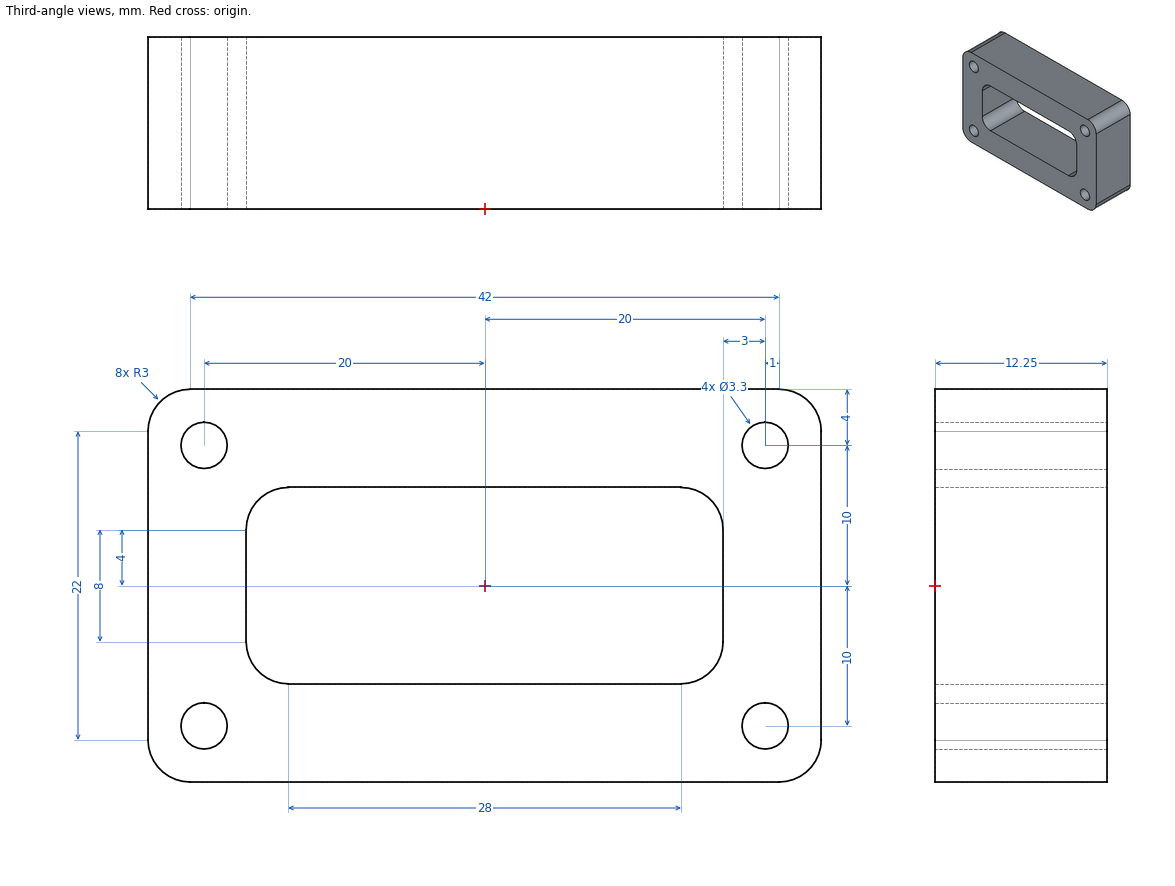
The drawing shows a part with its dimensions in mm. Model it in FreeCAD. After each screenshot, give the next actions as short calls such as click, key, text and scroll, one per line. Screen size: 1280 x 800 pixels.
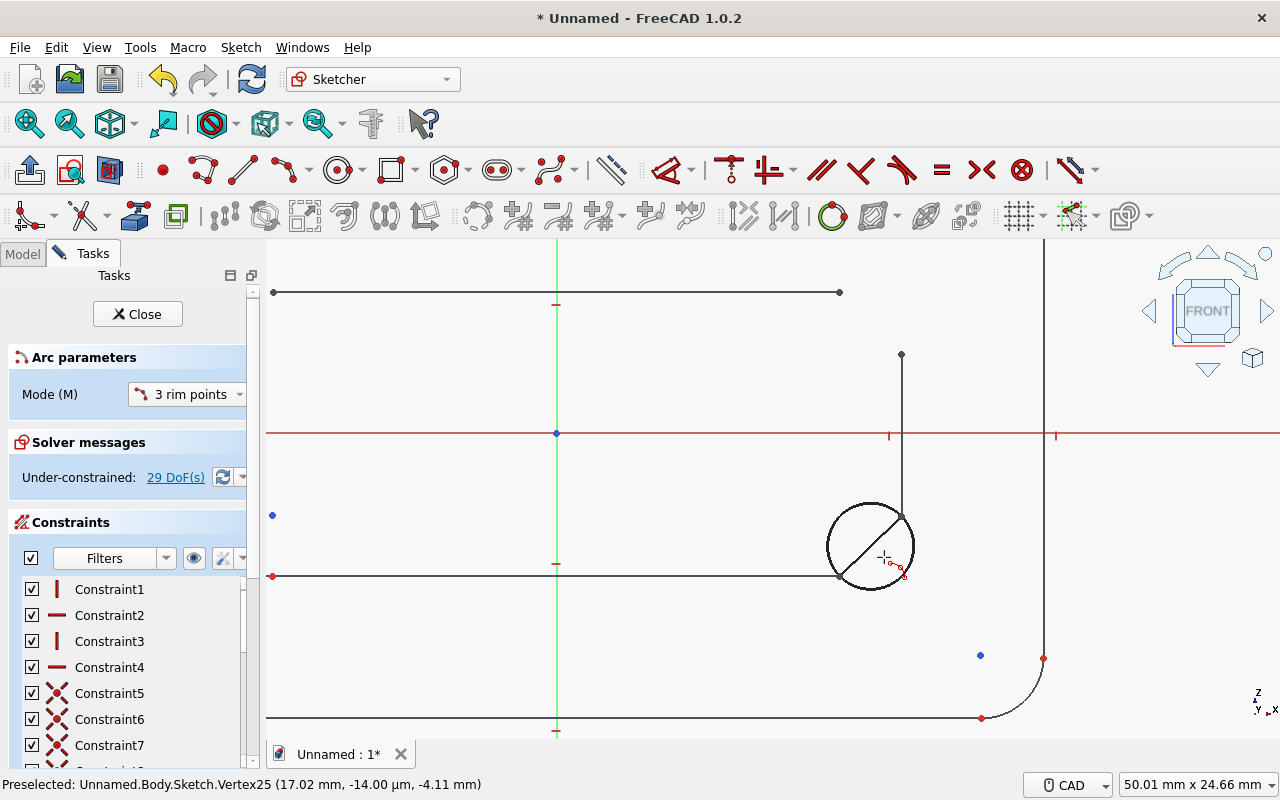
click(883, 557)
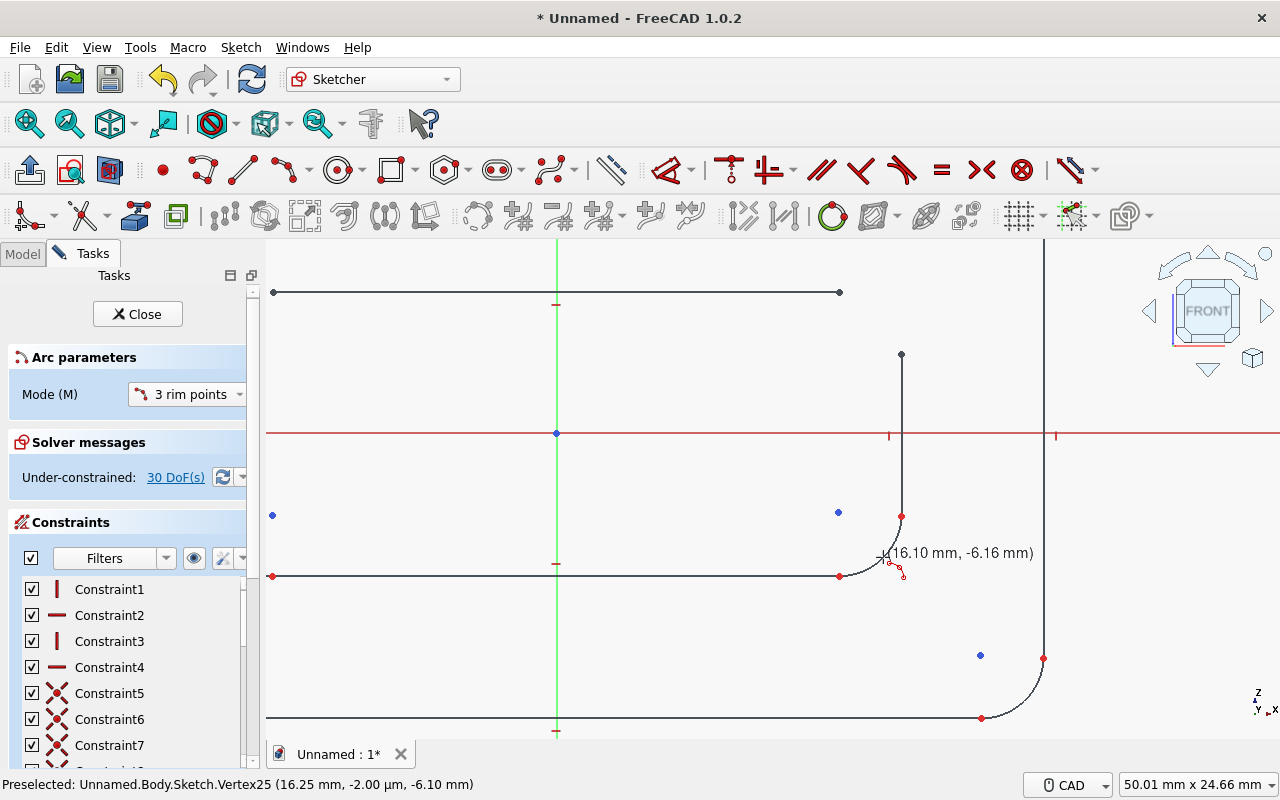
click(902, 354)
click(840, 292)
click(883, 309)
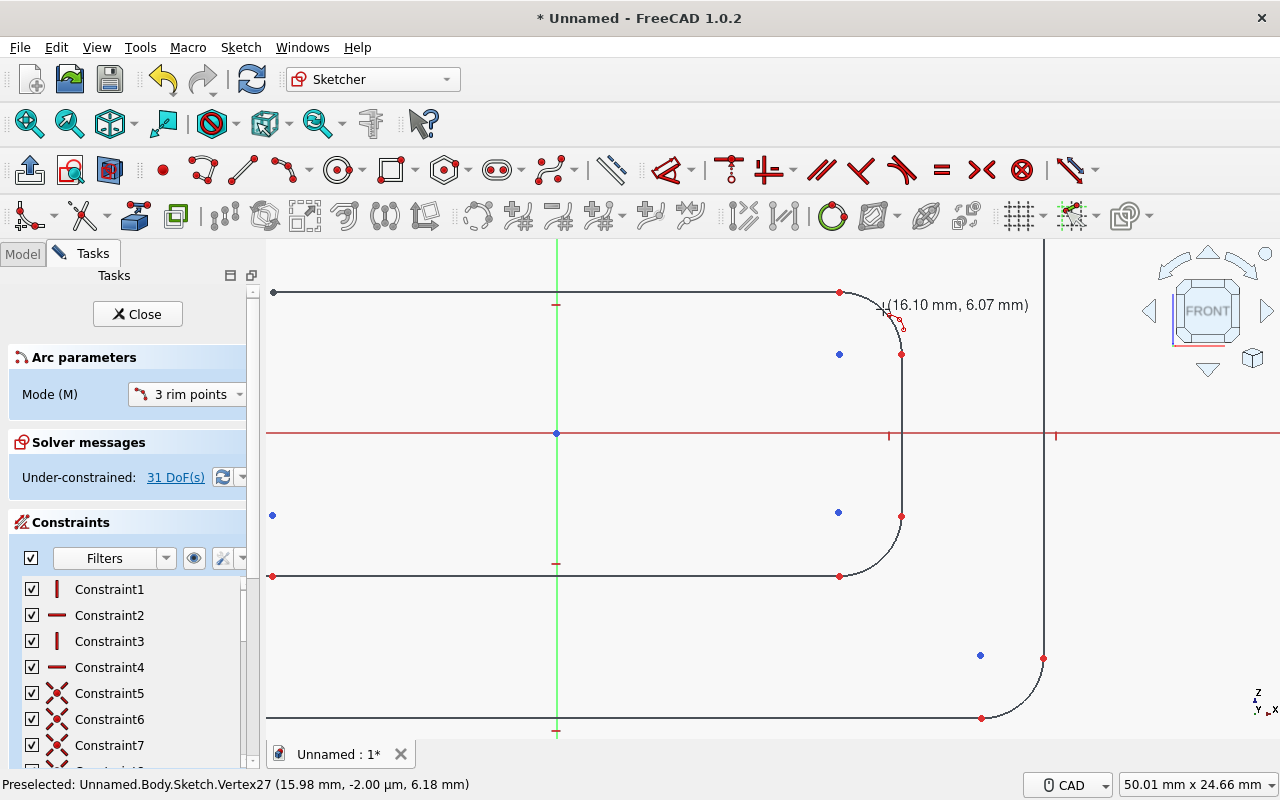
scroll(884, 557, down, 3)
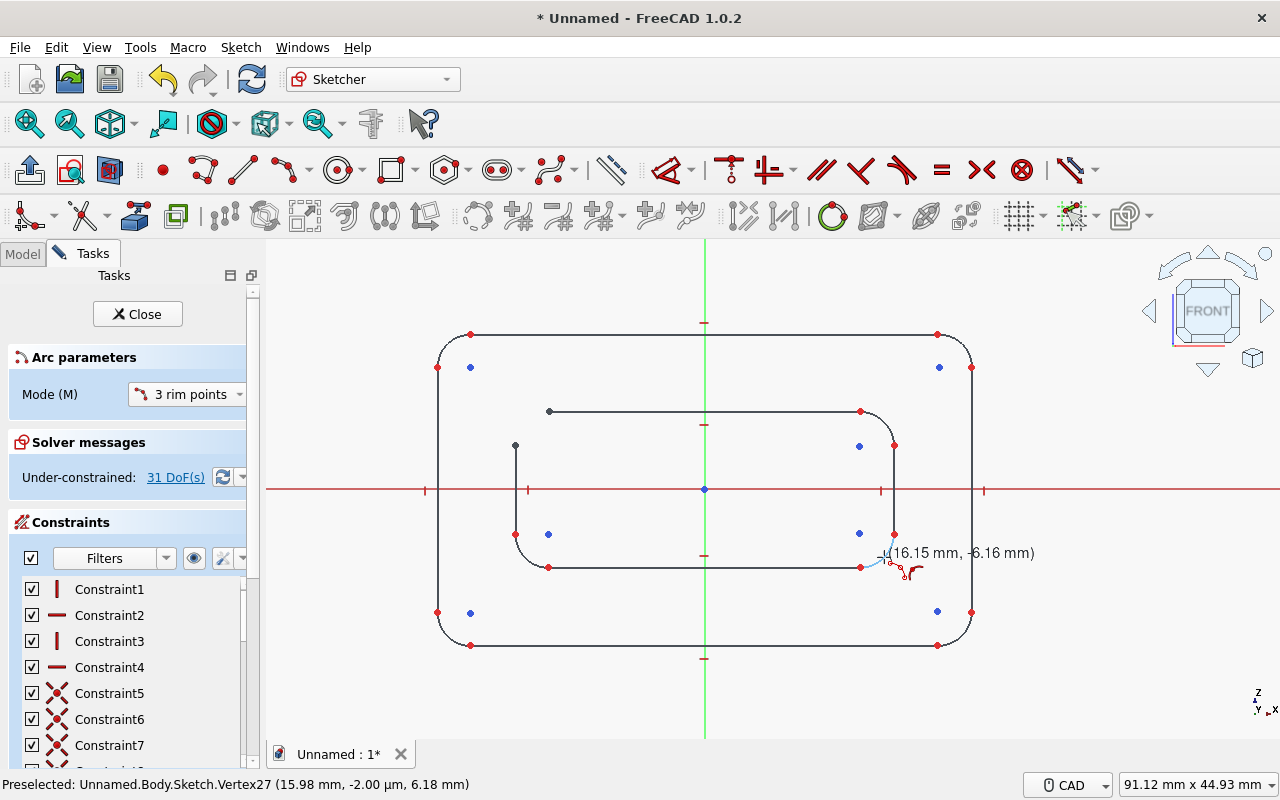
click(549, 412)
click(516, 445)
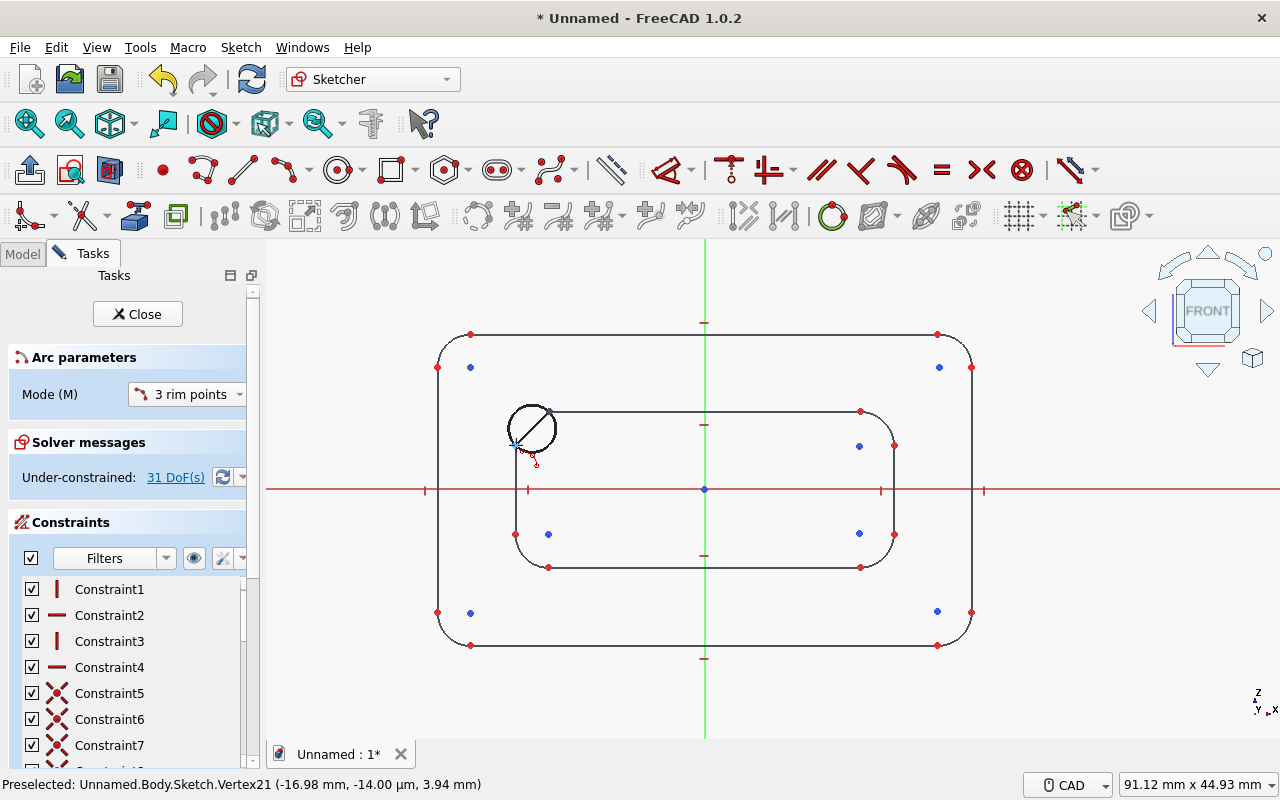
scroll(525, 421, up, 3)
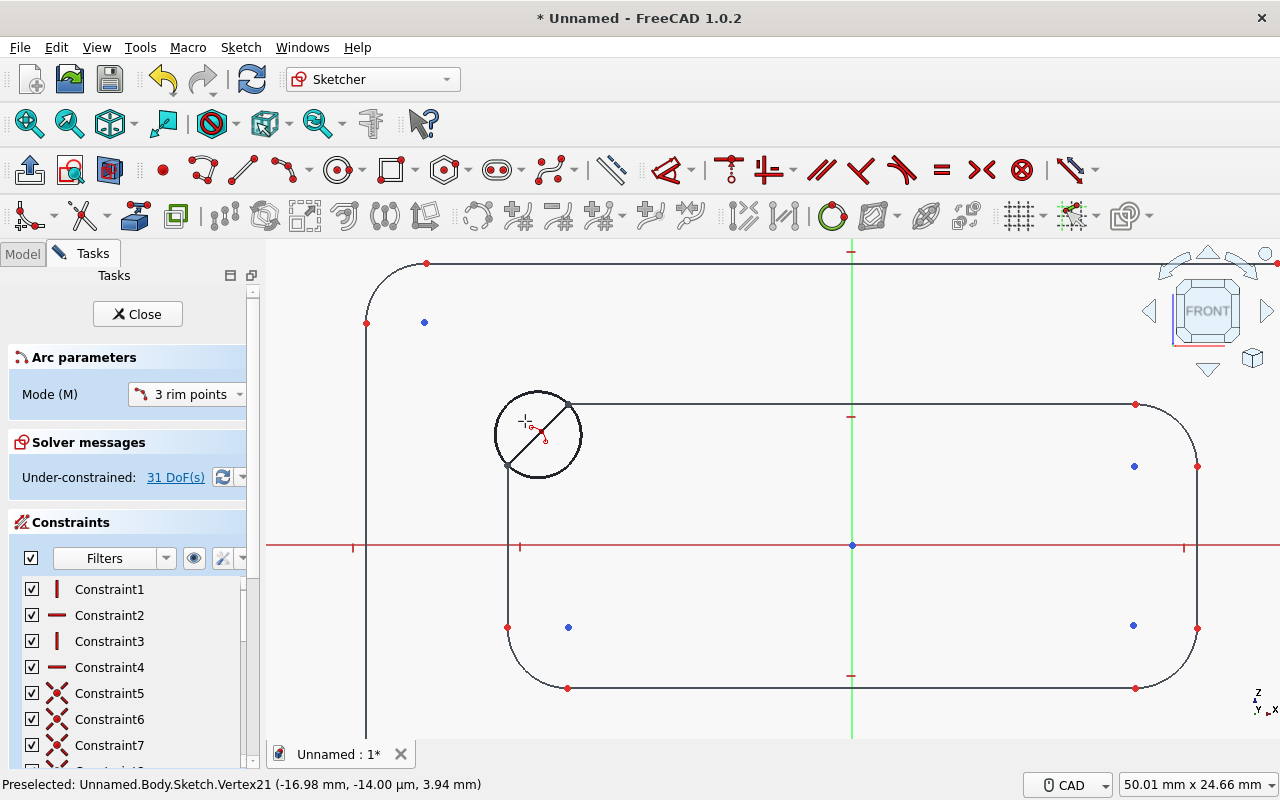
click(525, 421)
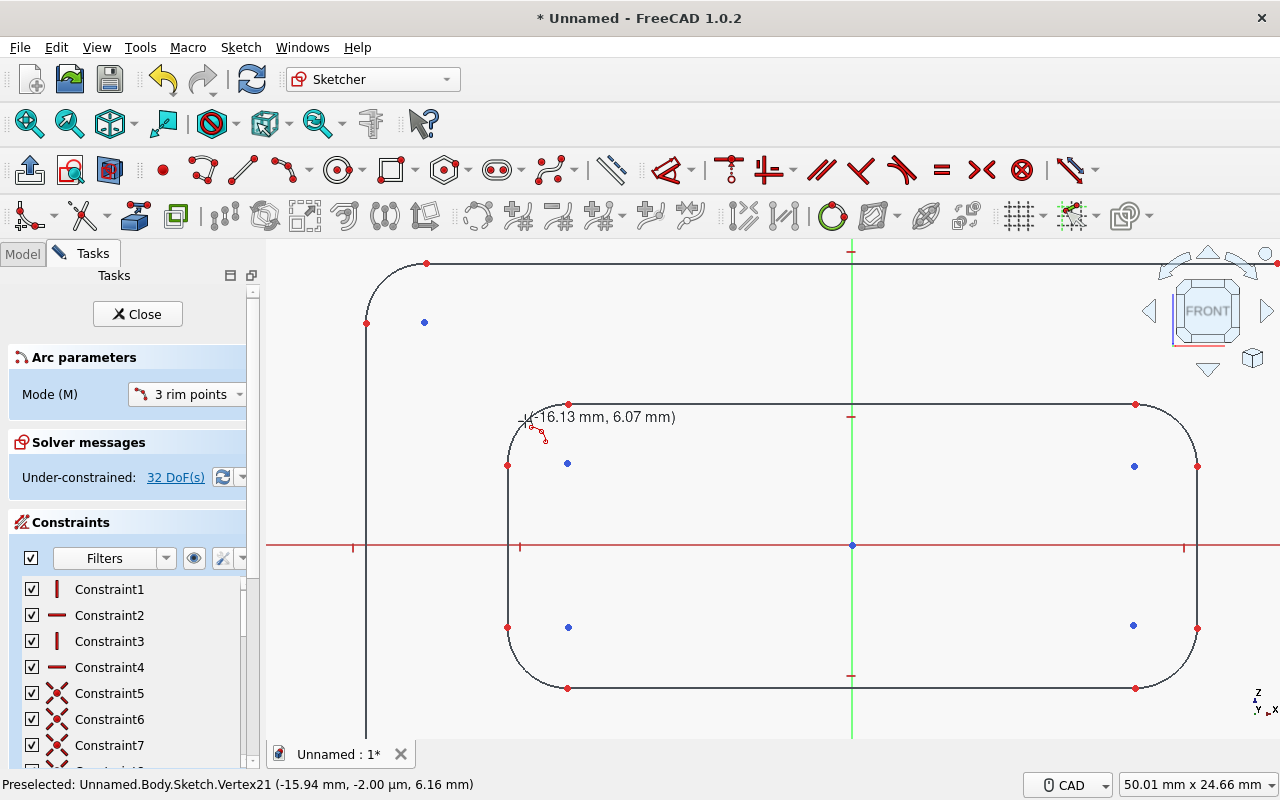
click(338, 170)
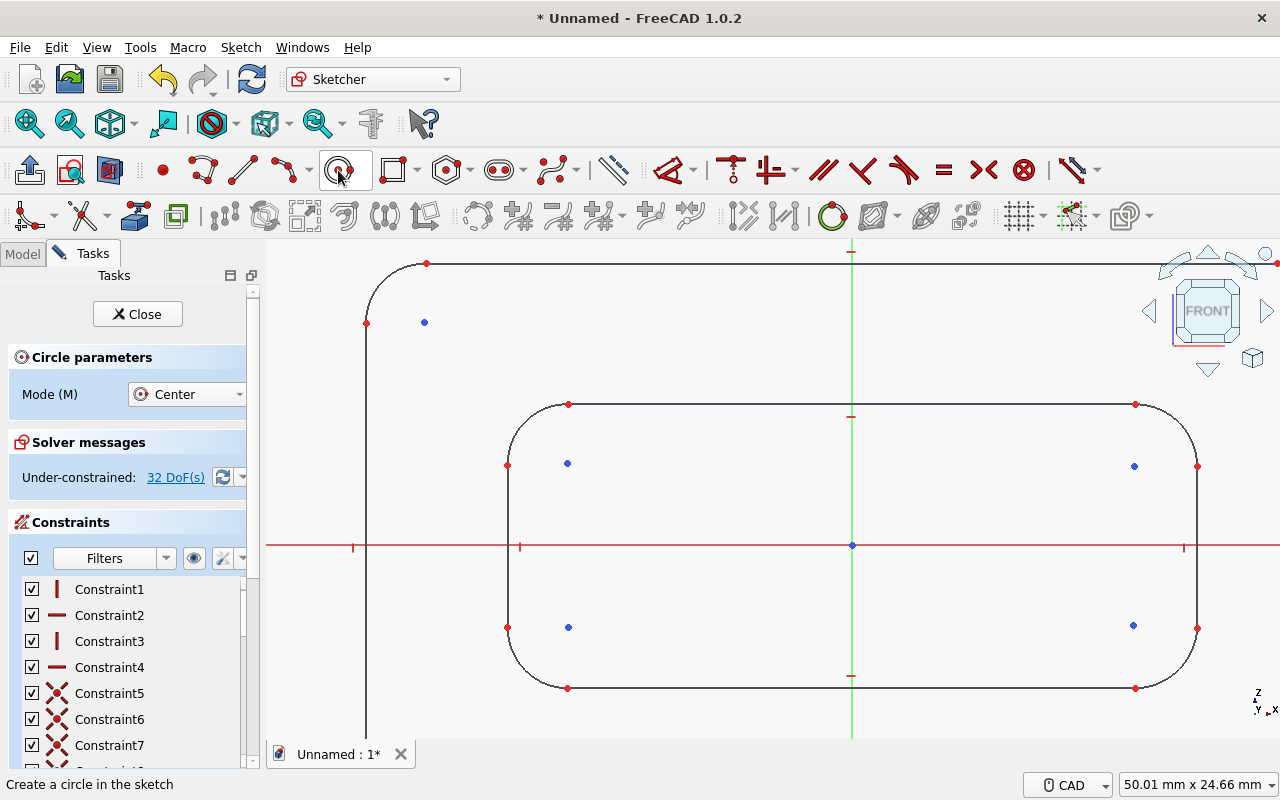
scroll(525, 421, down, 3)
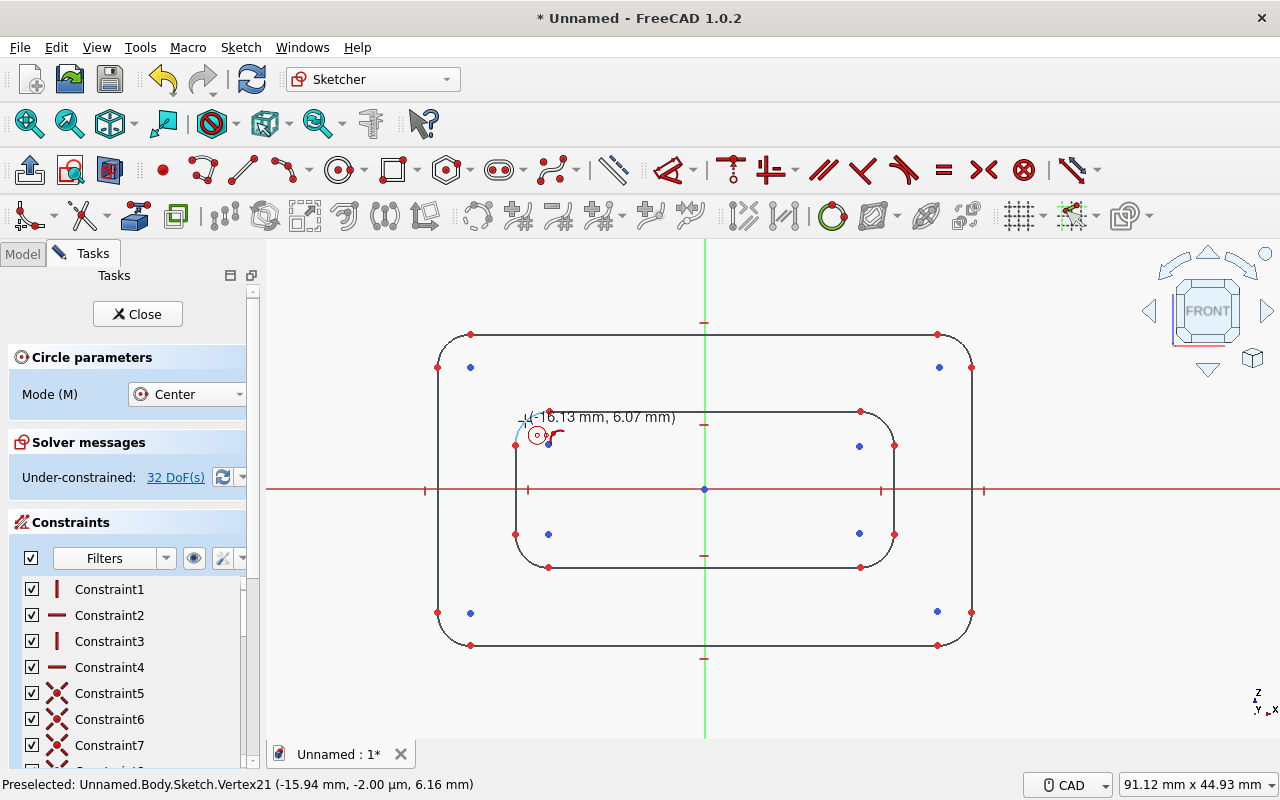
scroll(927, 378, up, 2)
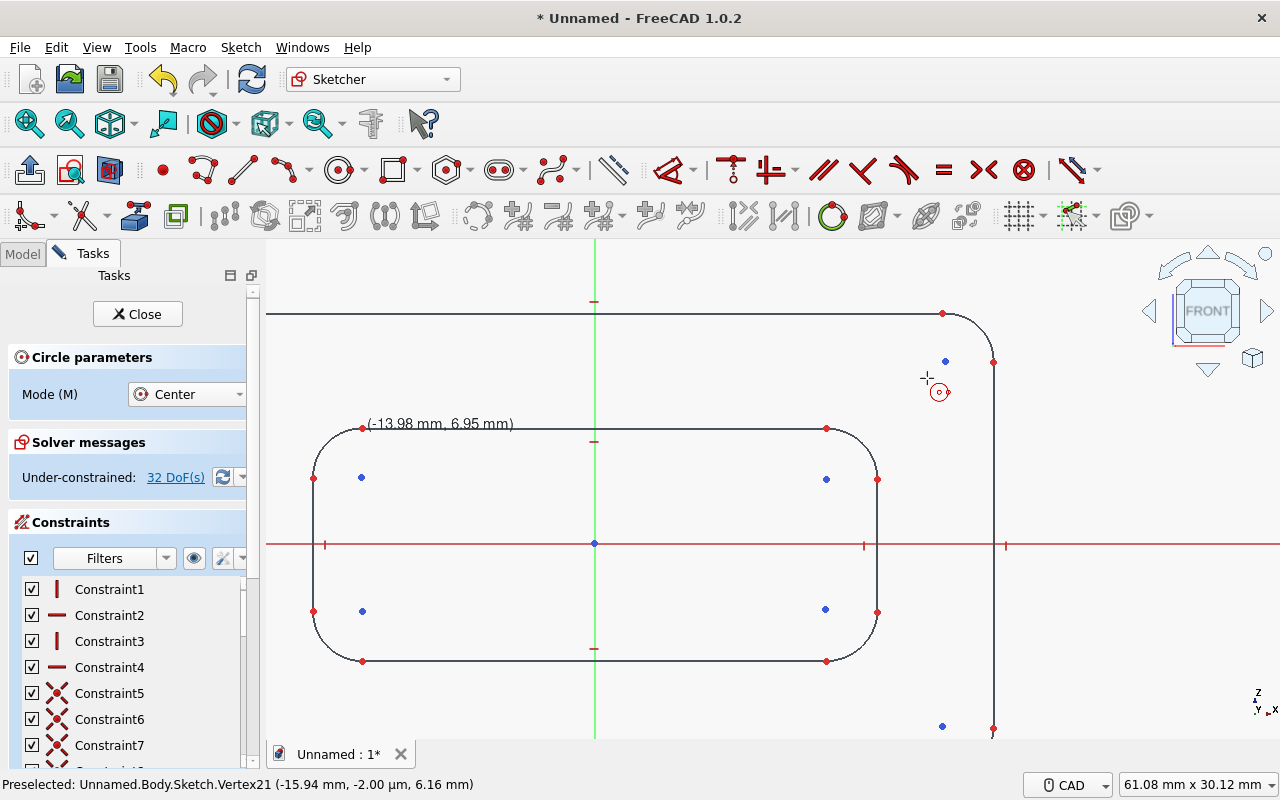
click(927, 378)
click(908, 359)